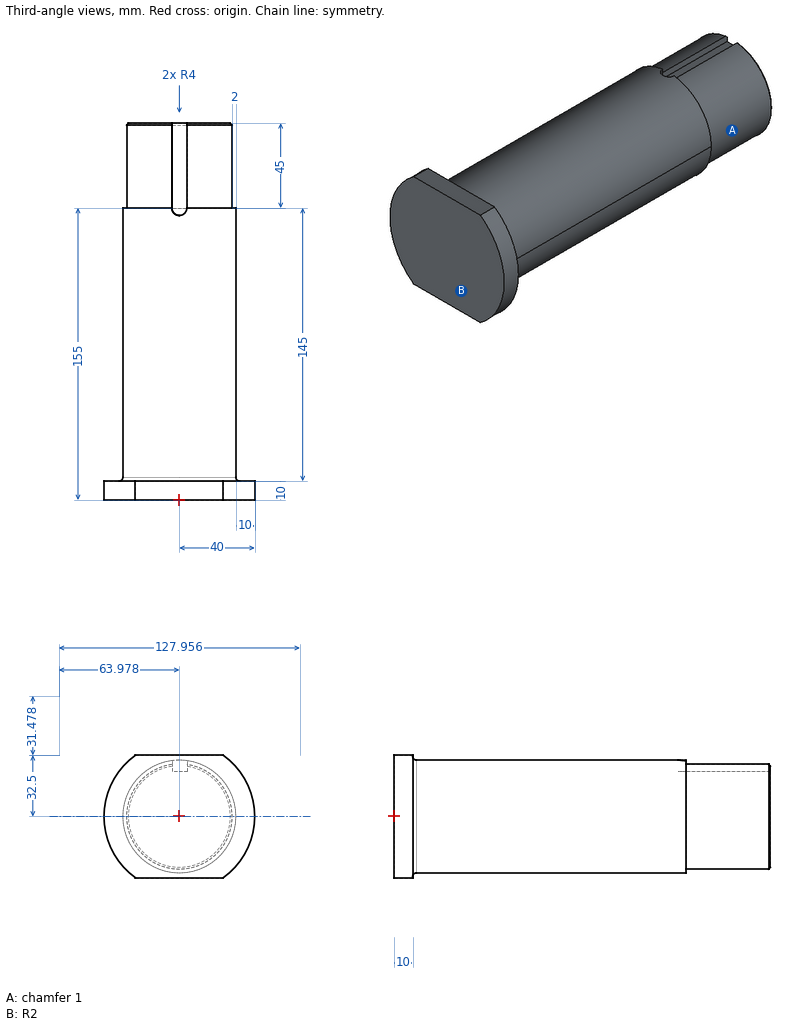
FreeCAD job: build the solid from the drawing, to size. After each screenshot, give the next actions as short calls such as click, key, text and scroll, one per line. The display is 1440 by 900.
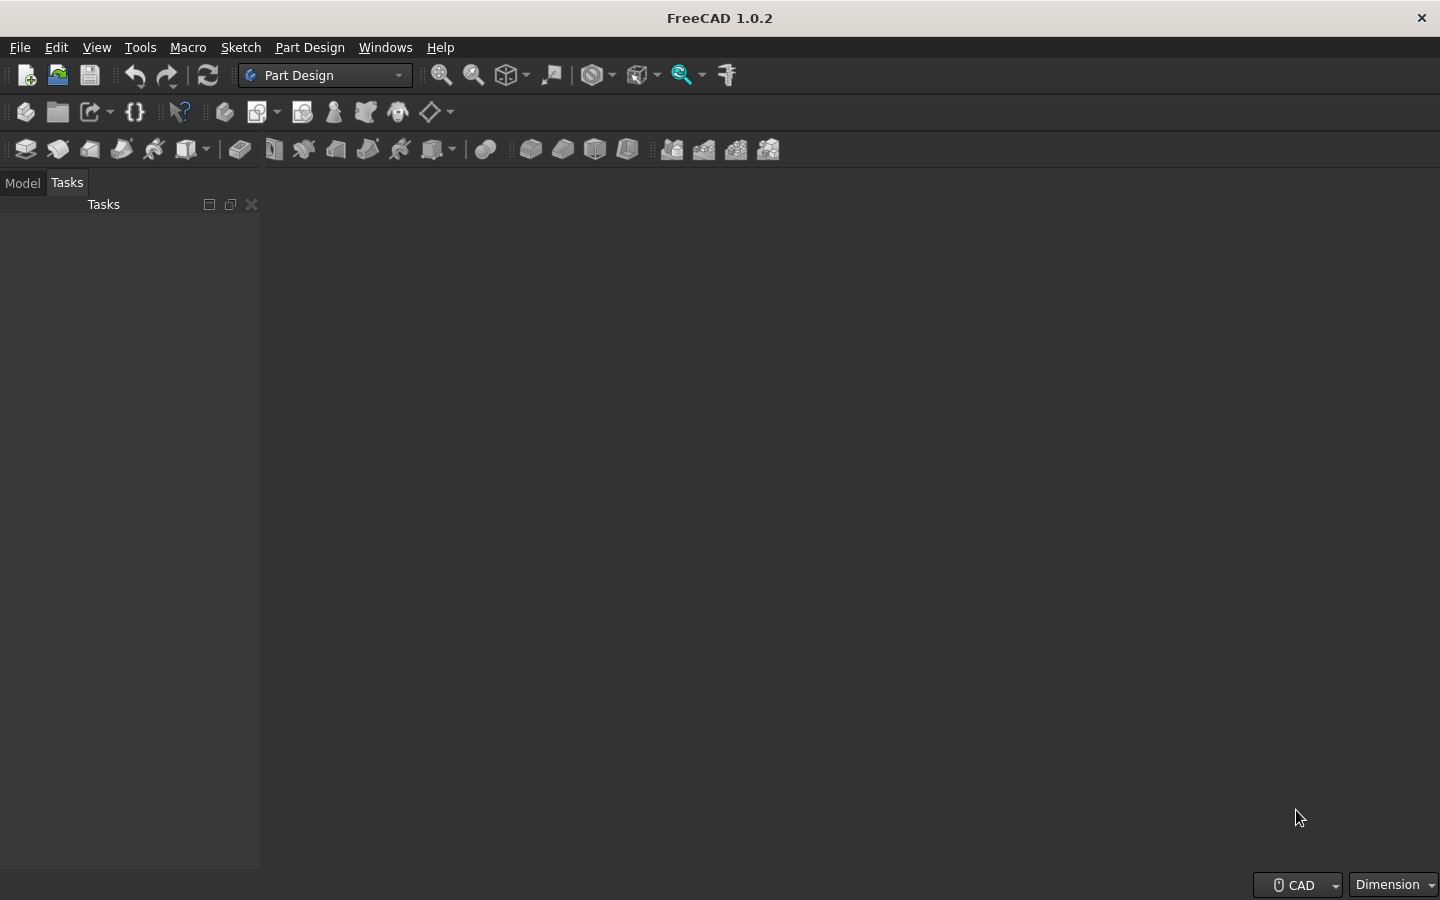
click(414, 76)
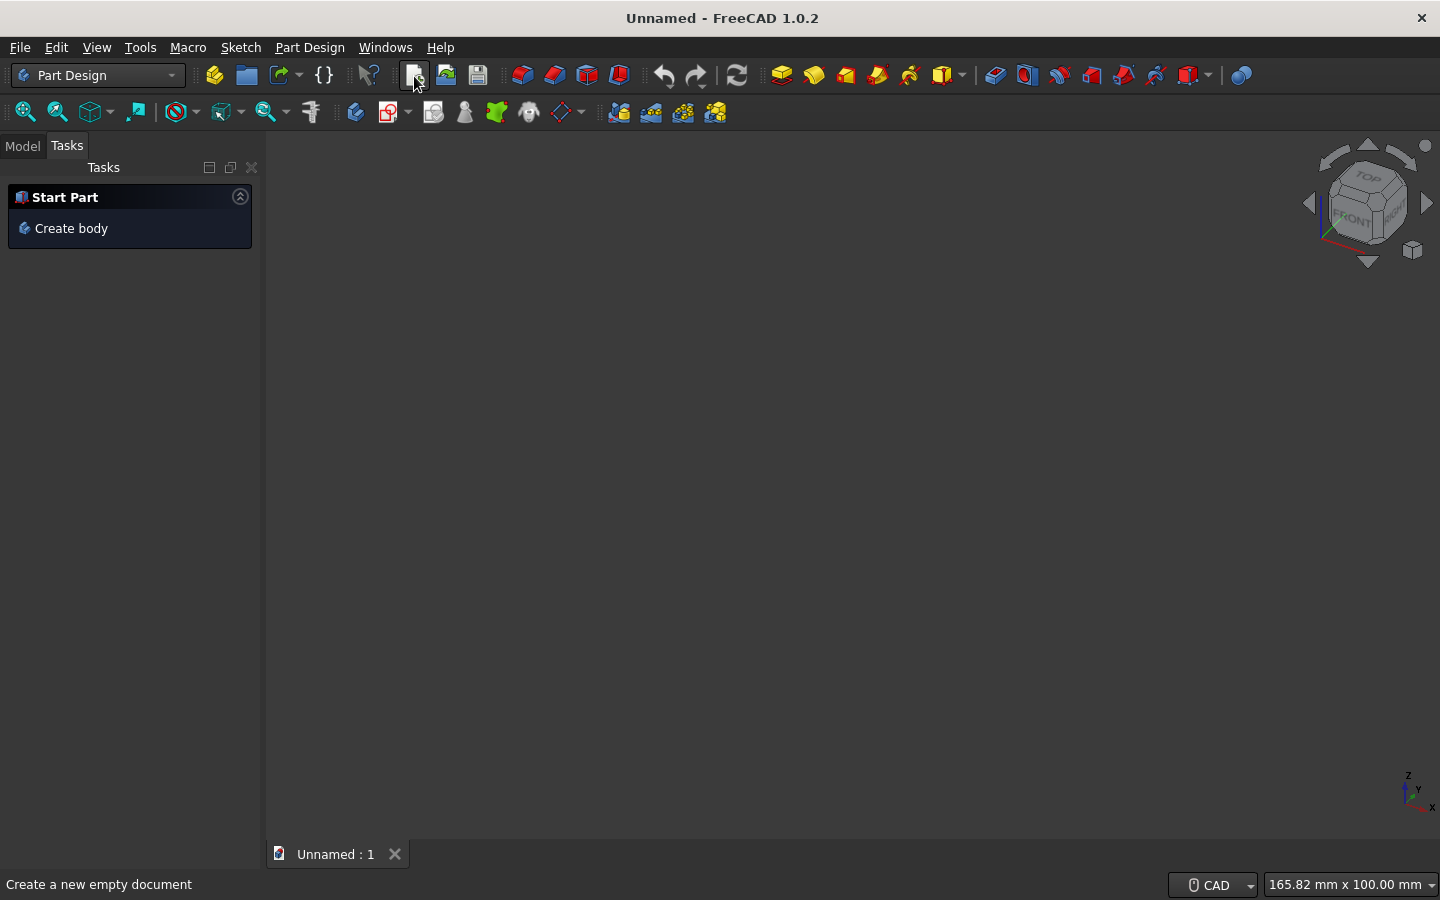
click(388, 112)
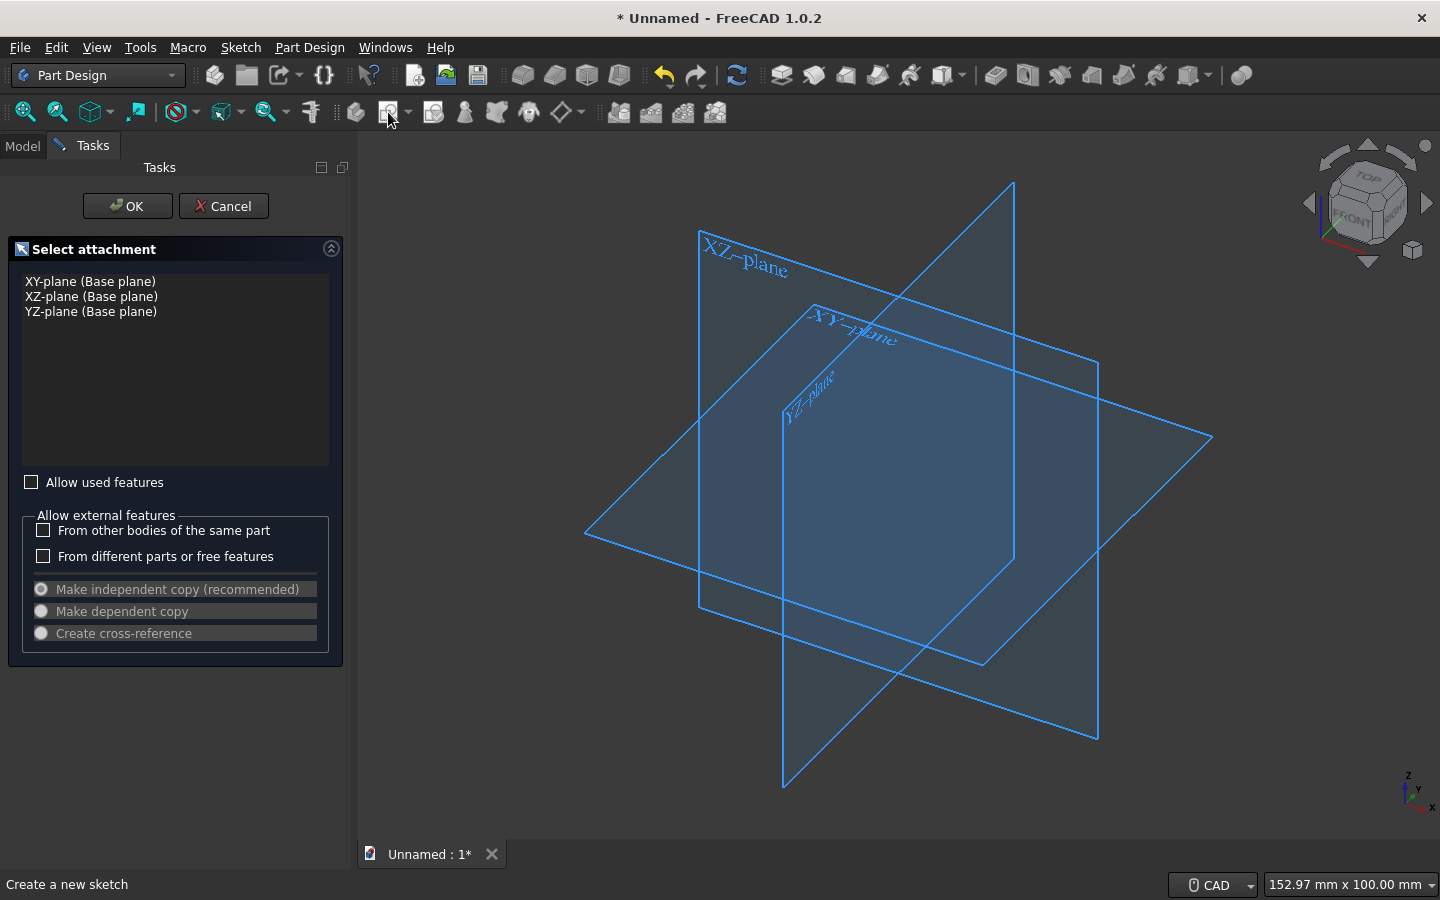
click(82, 282)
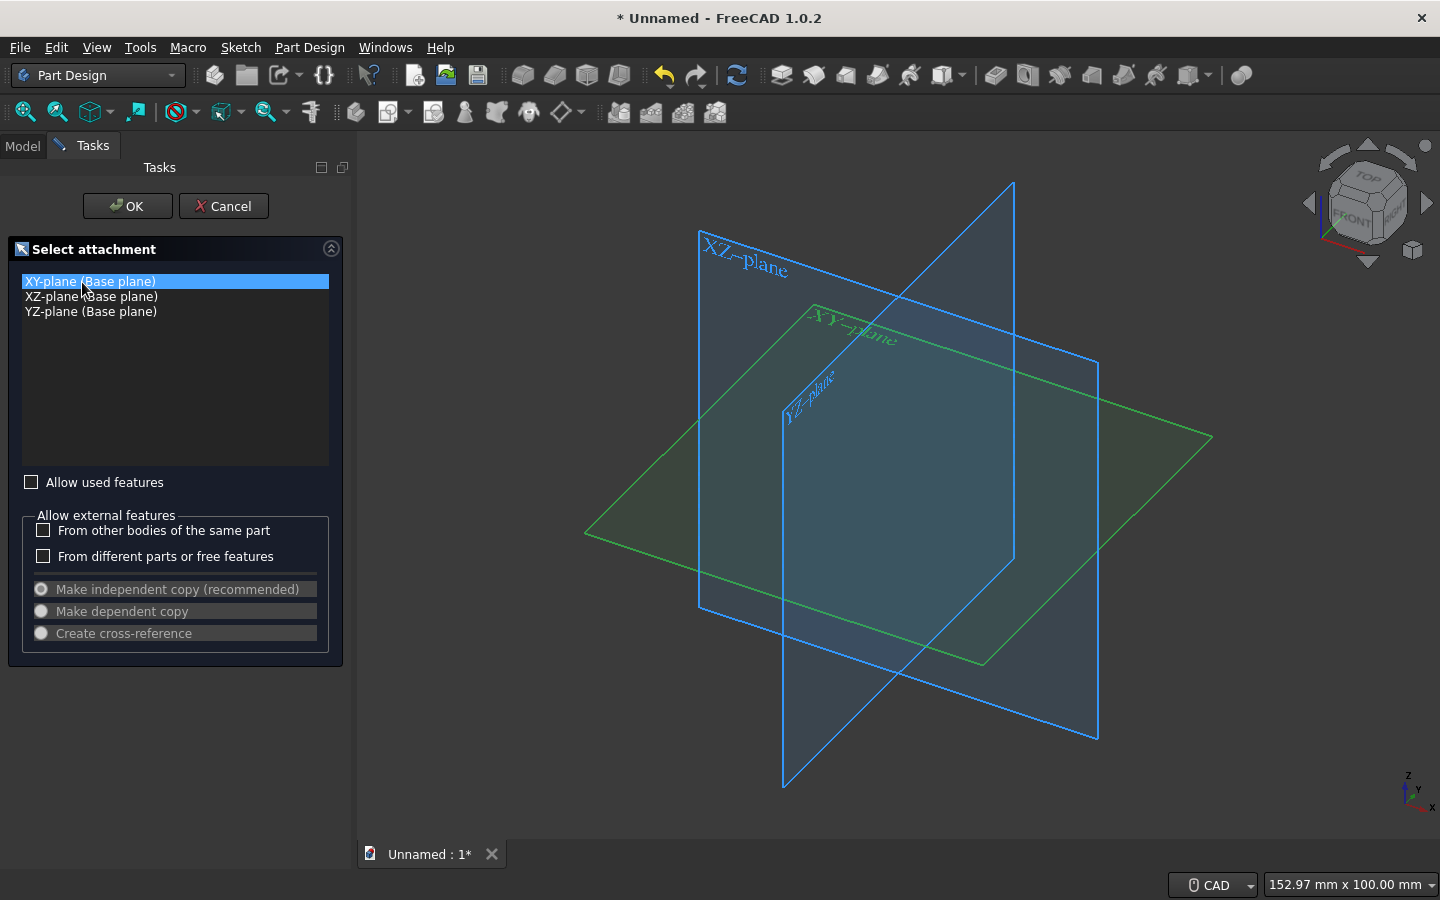
click(128, 206)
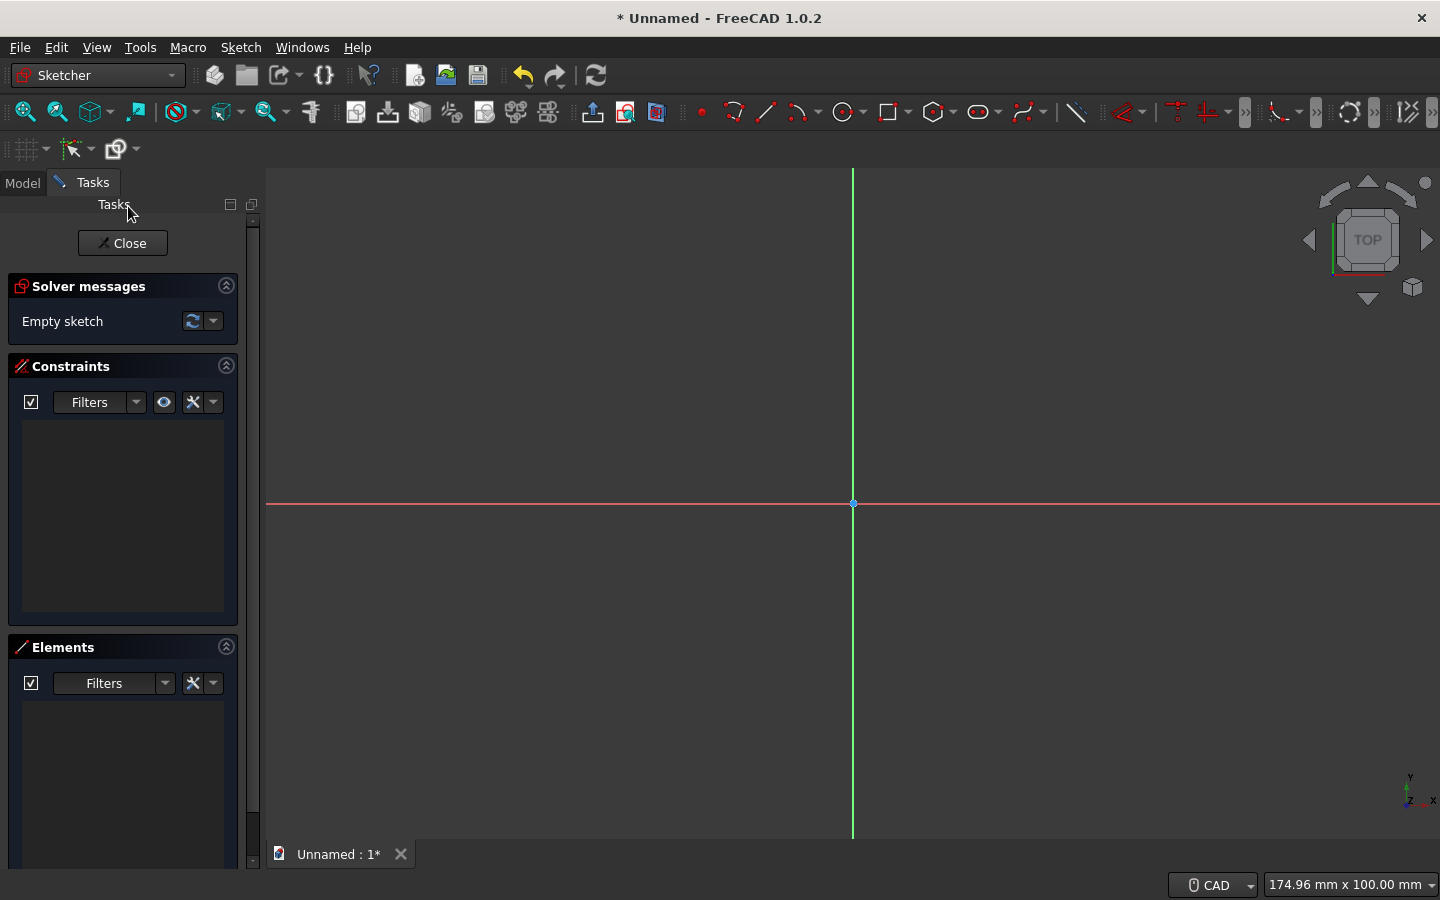
scroll(697, 793, down, 6)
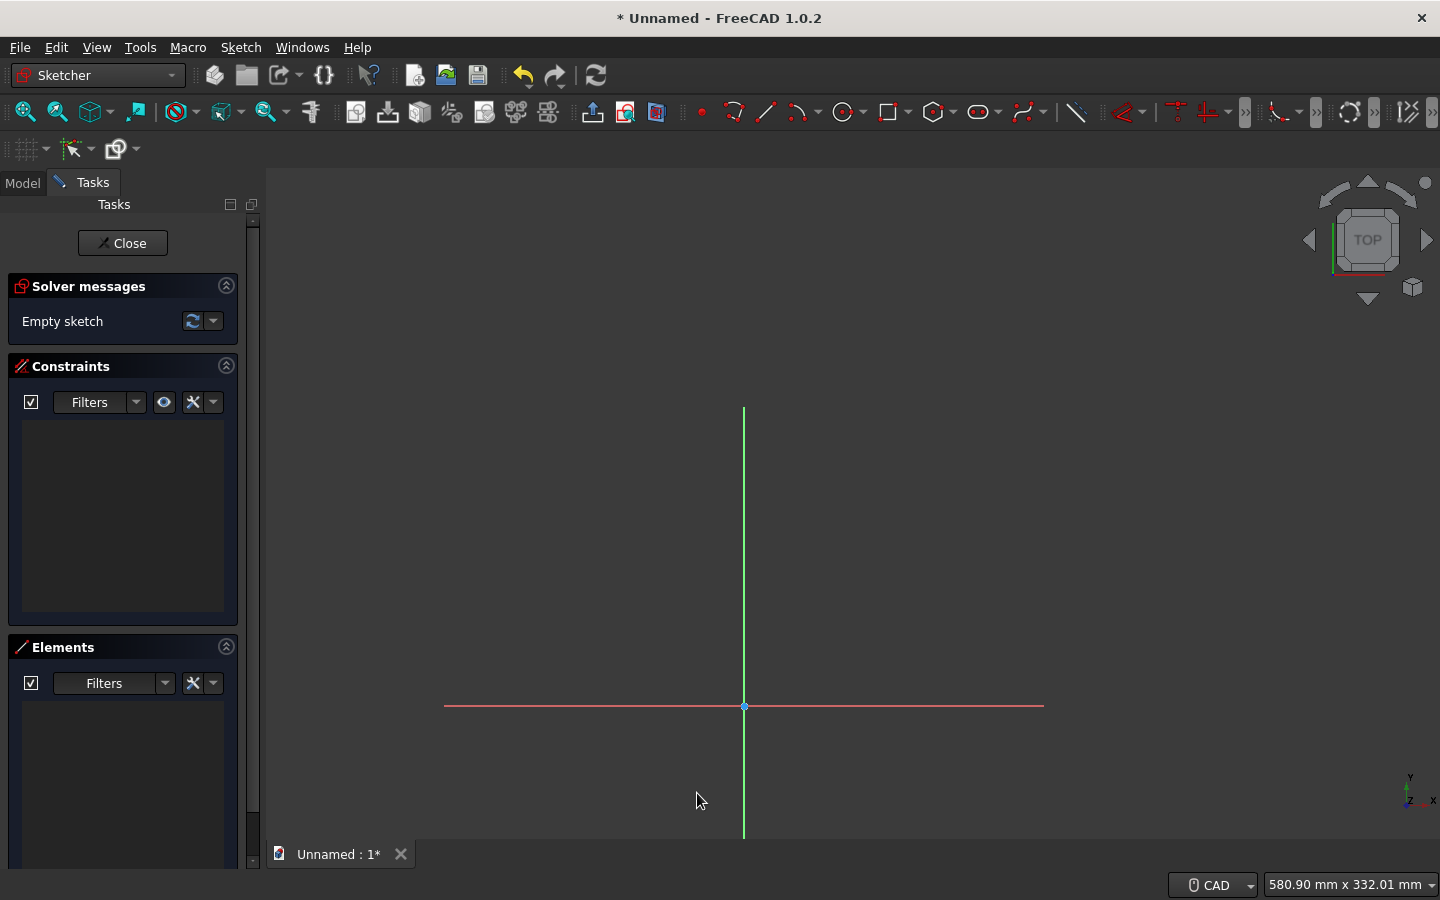
click(734, 112)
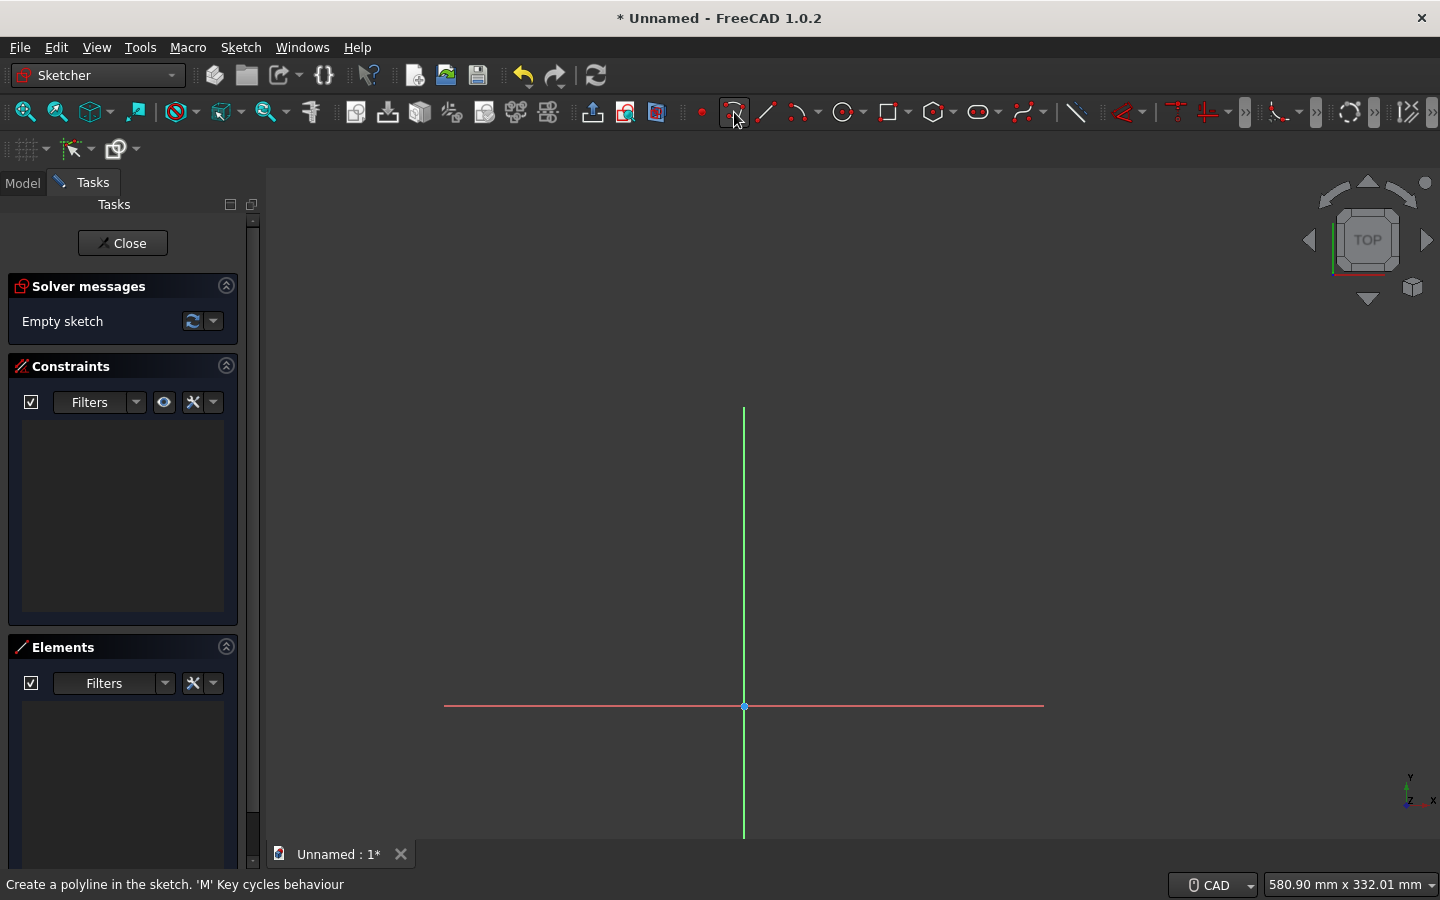
click(744, 706)
click(825, 697)
click(825, 686)
click(805, 686)
click(805, 393)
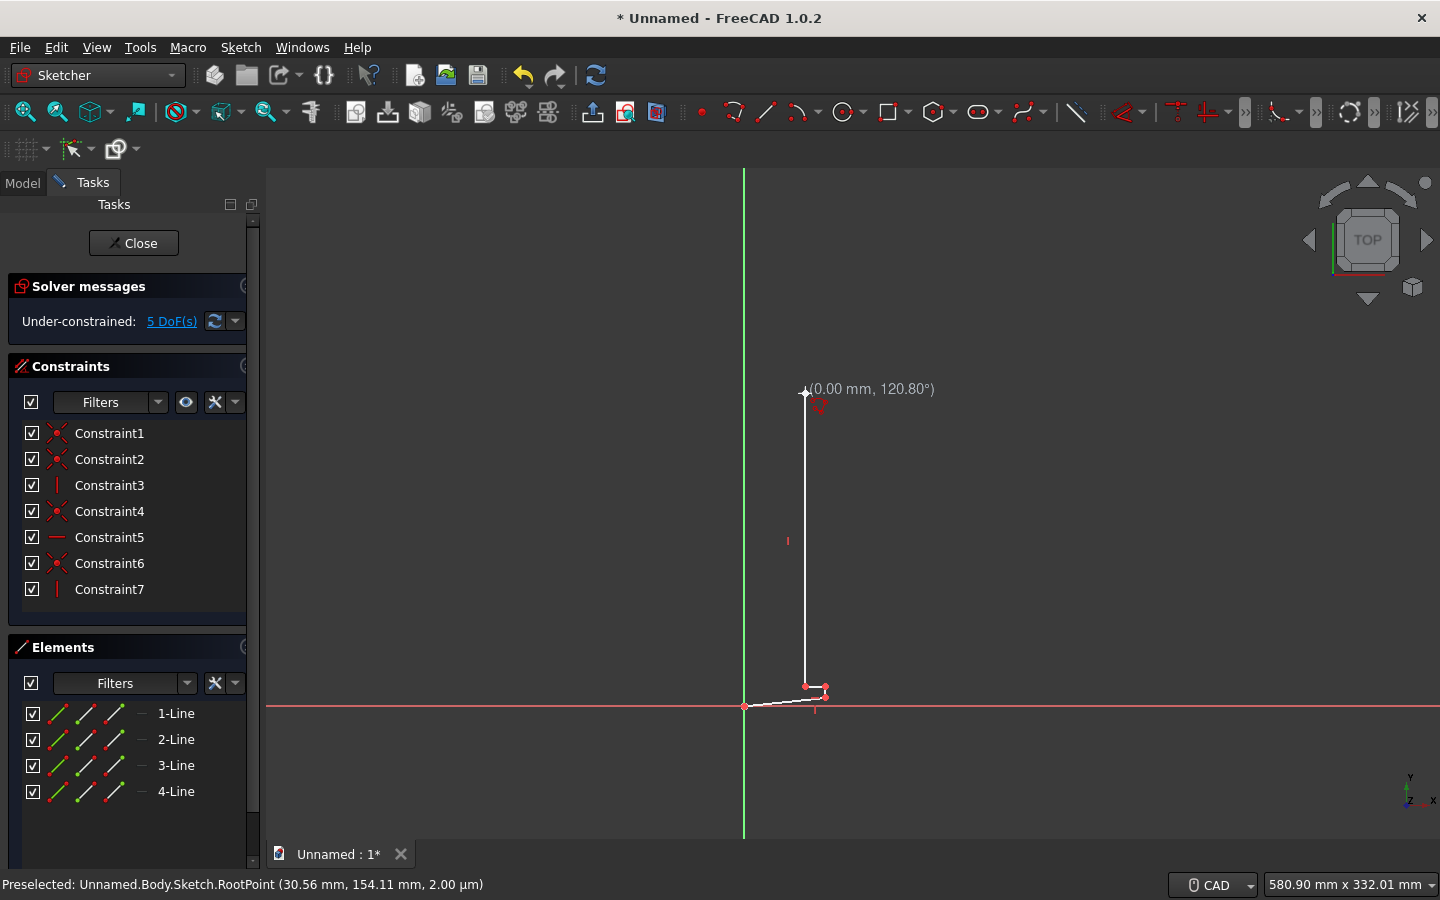
scroll(801, 393, up, 7)